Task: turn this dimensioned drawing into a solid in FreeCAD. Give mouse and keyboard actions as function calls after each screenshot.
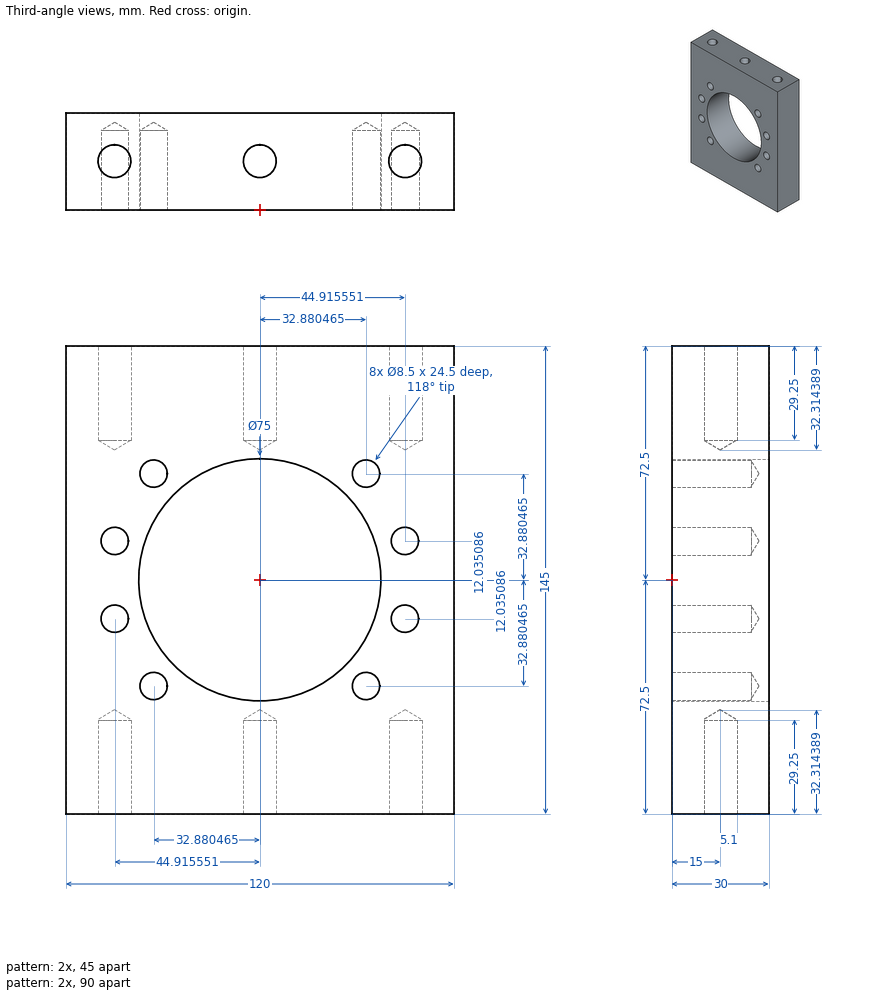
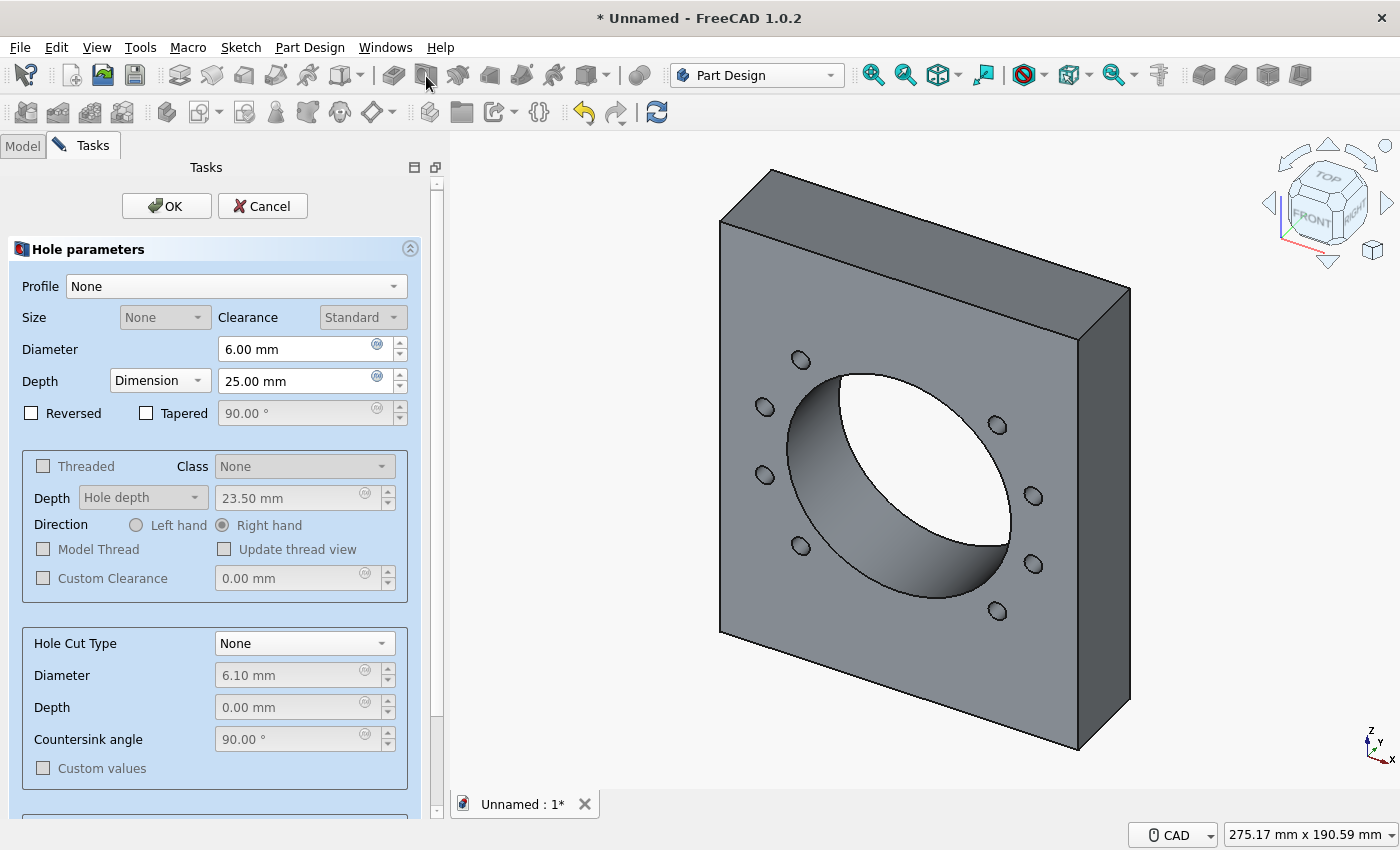
triple_click(305, 349)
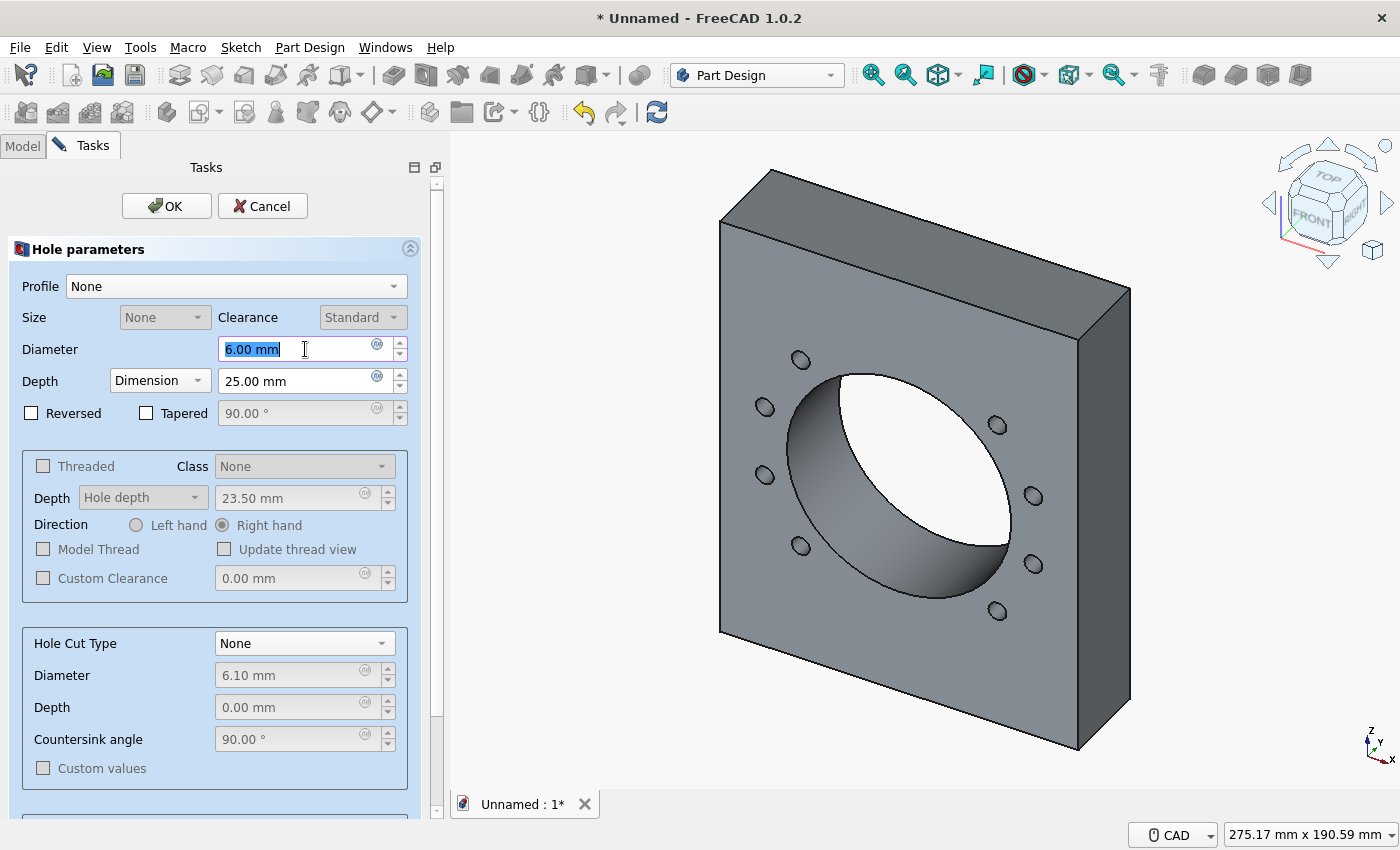
text(8.5)
key(Tab)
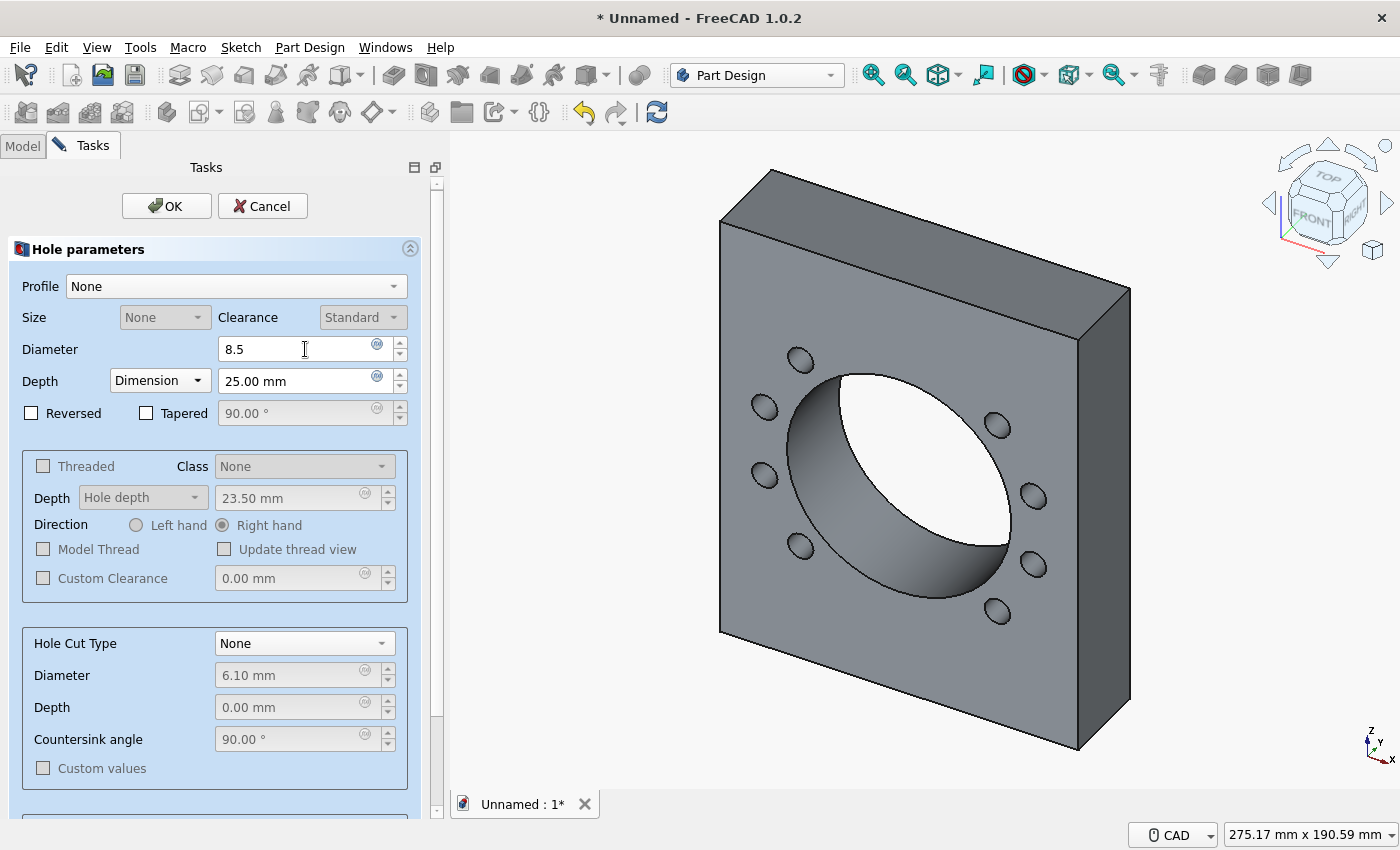
triple_click(305, 381)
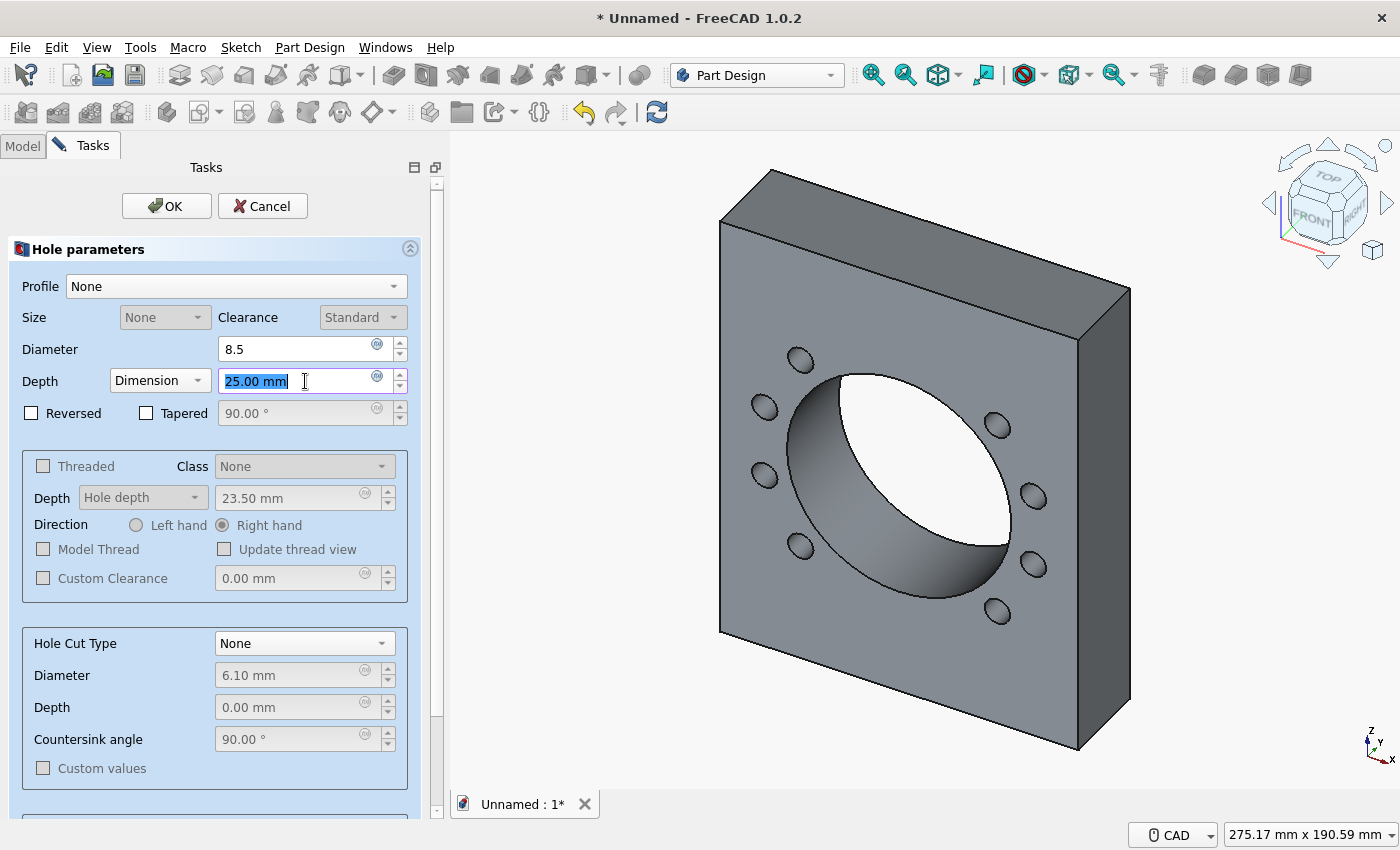
text(24.5)
key(Tab)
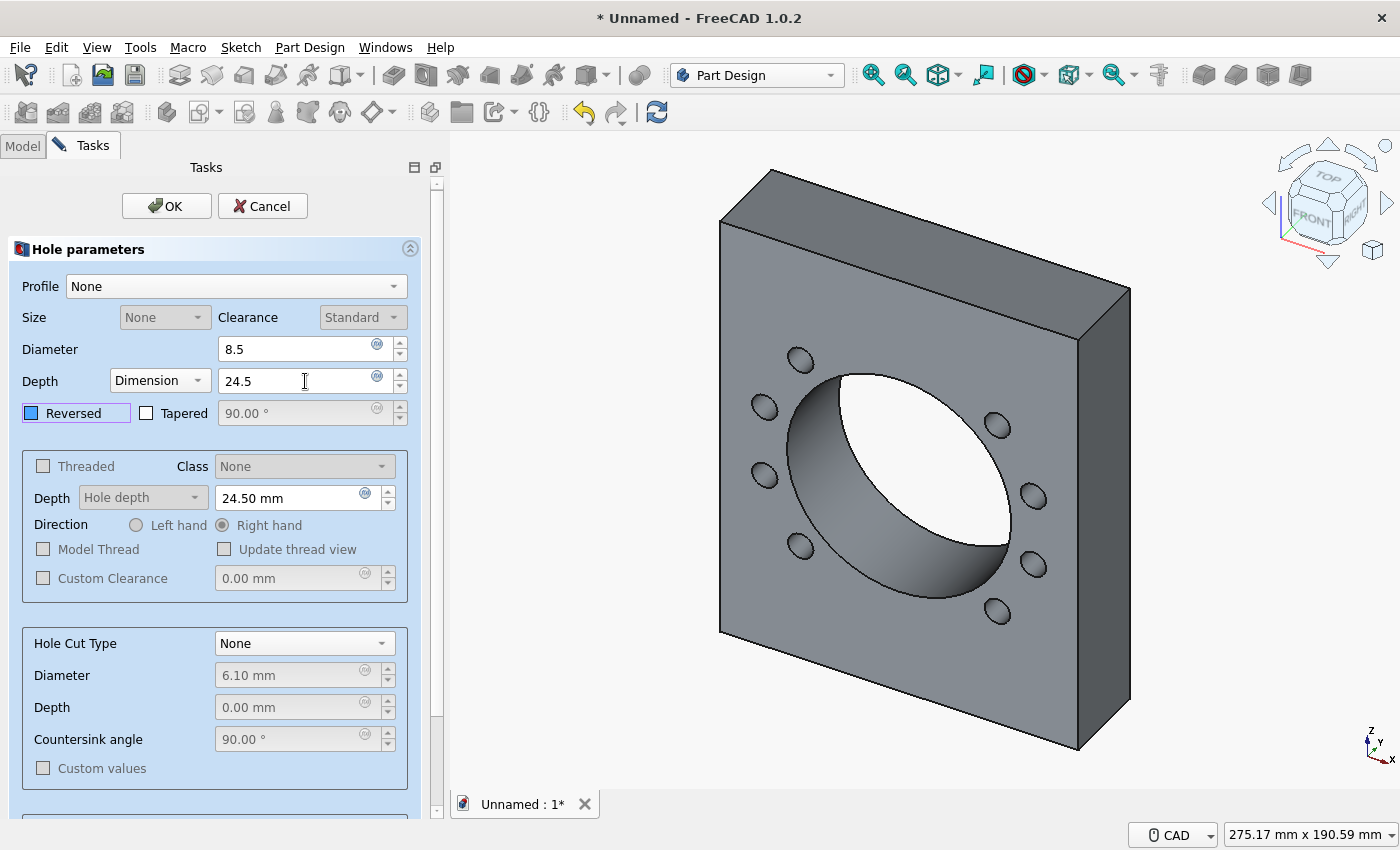
click(167, 206)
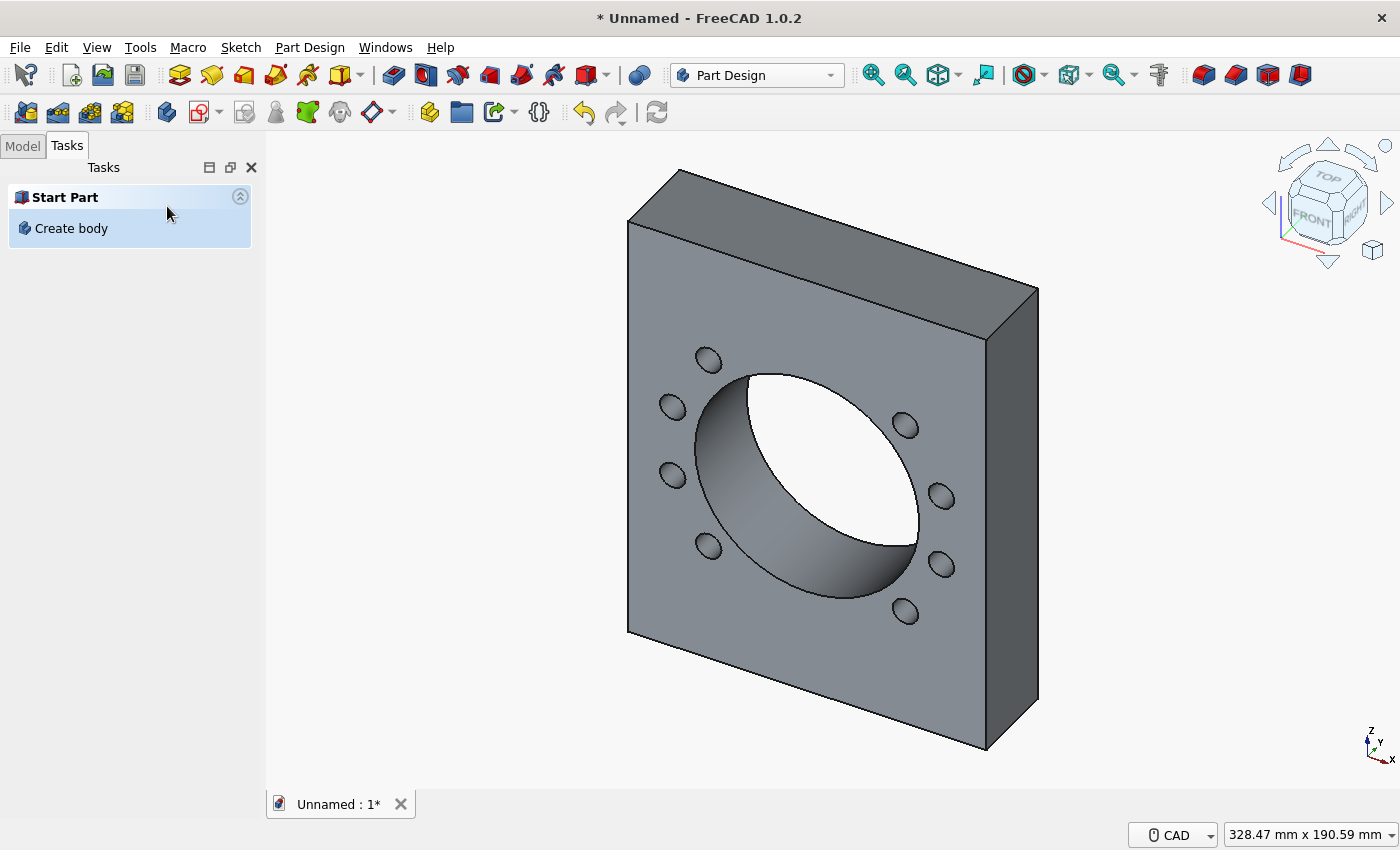
click(23, 145)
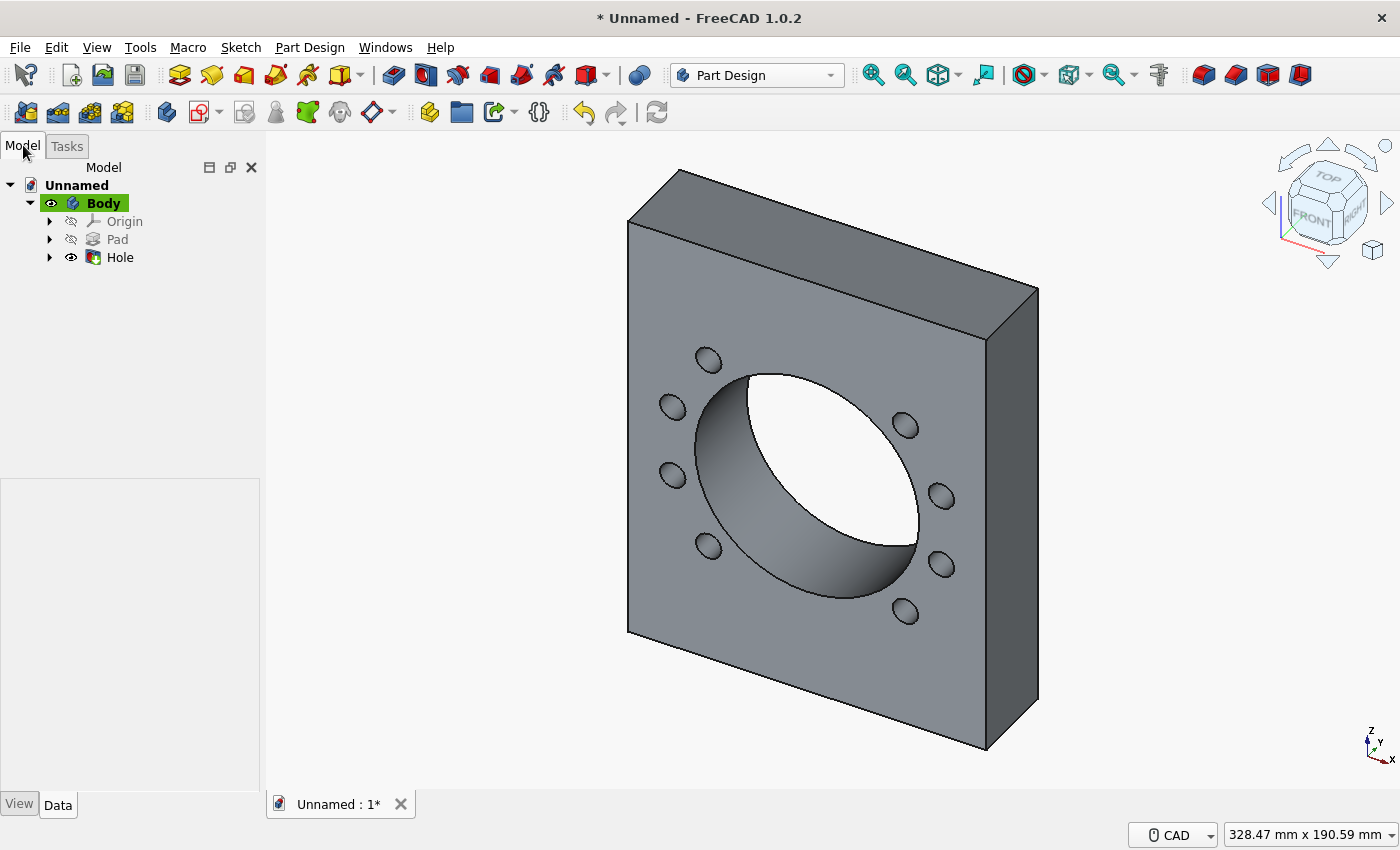
click(50, 221)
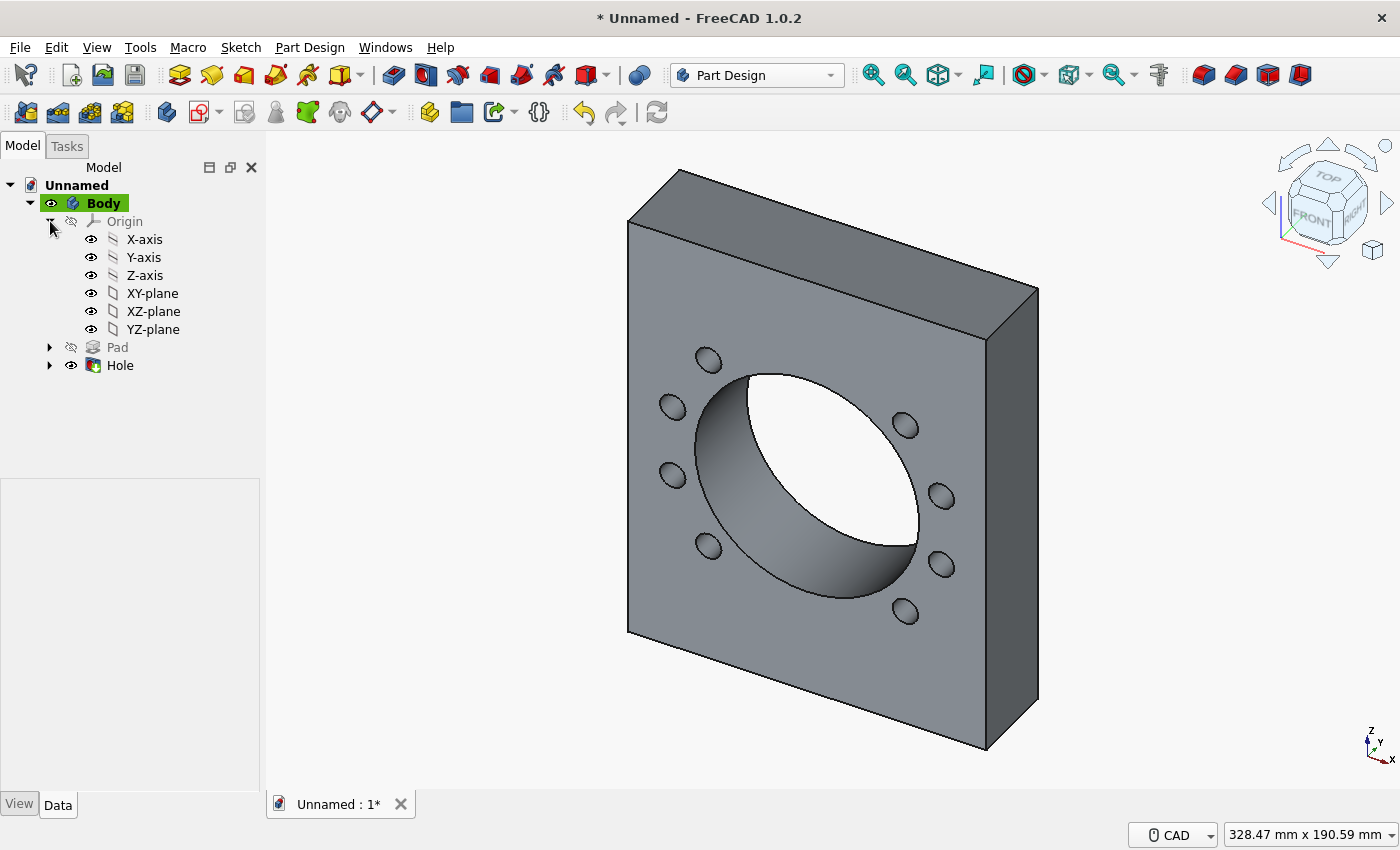
click(136, 329)